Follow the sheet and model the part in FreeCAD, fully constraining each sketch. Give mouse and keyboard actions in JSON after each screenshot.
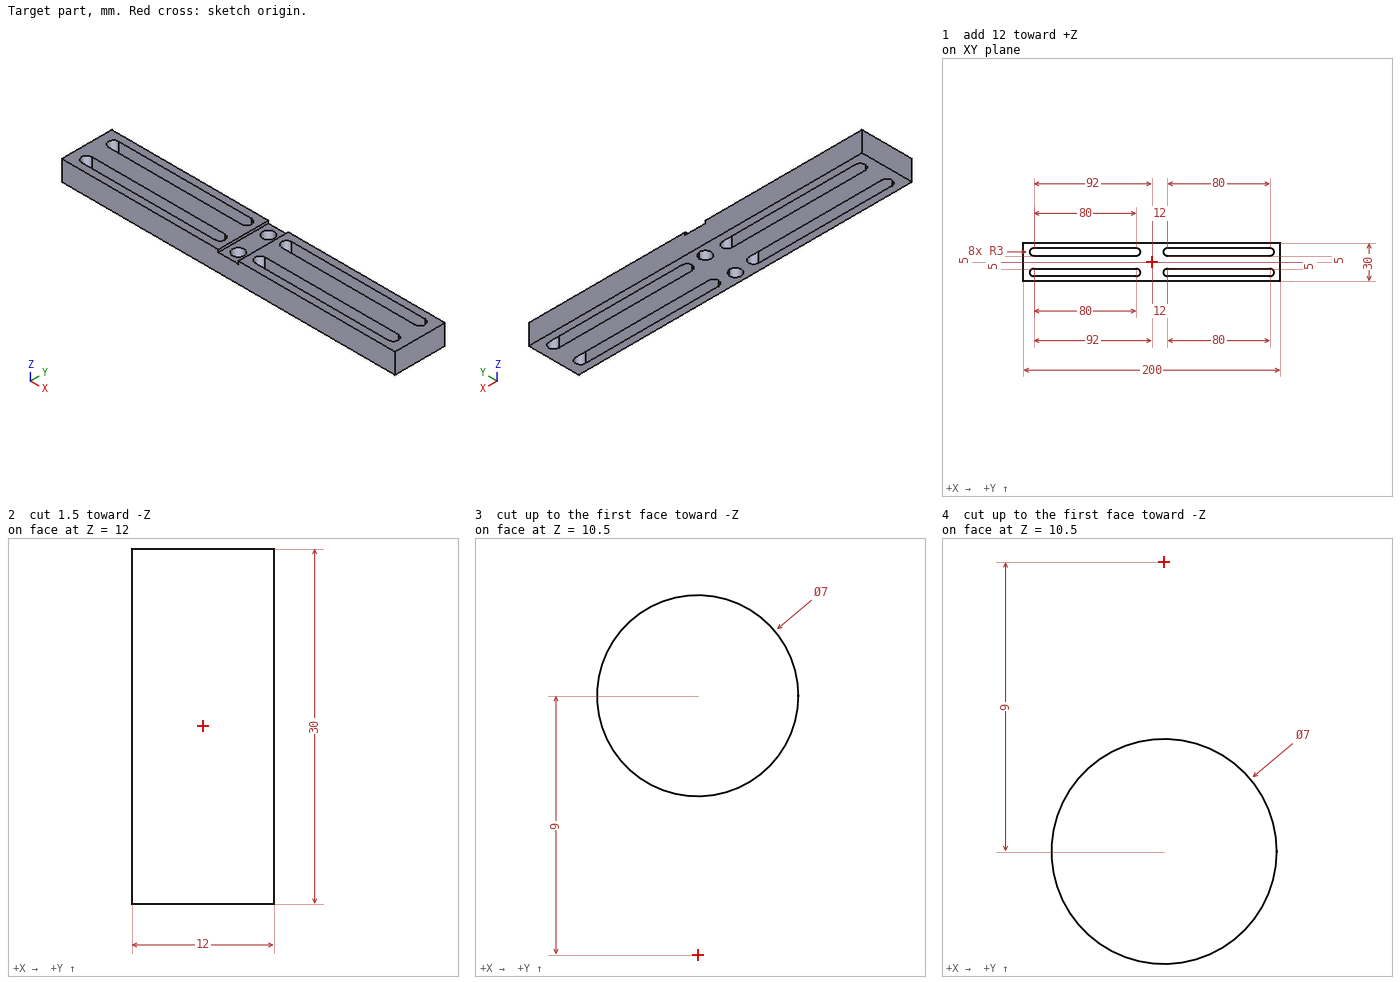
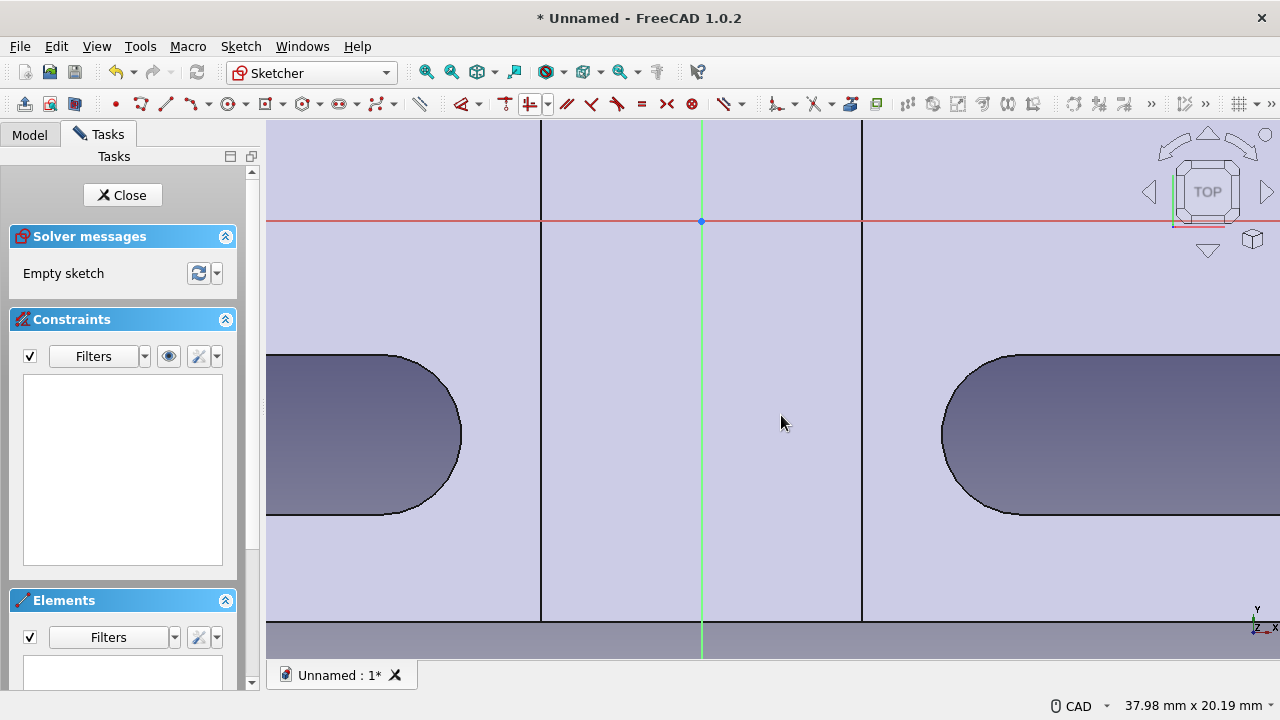
{"action": "left_click", "coordinate": [228, 104]}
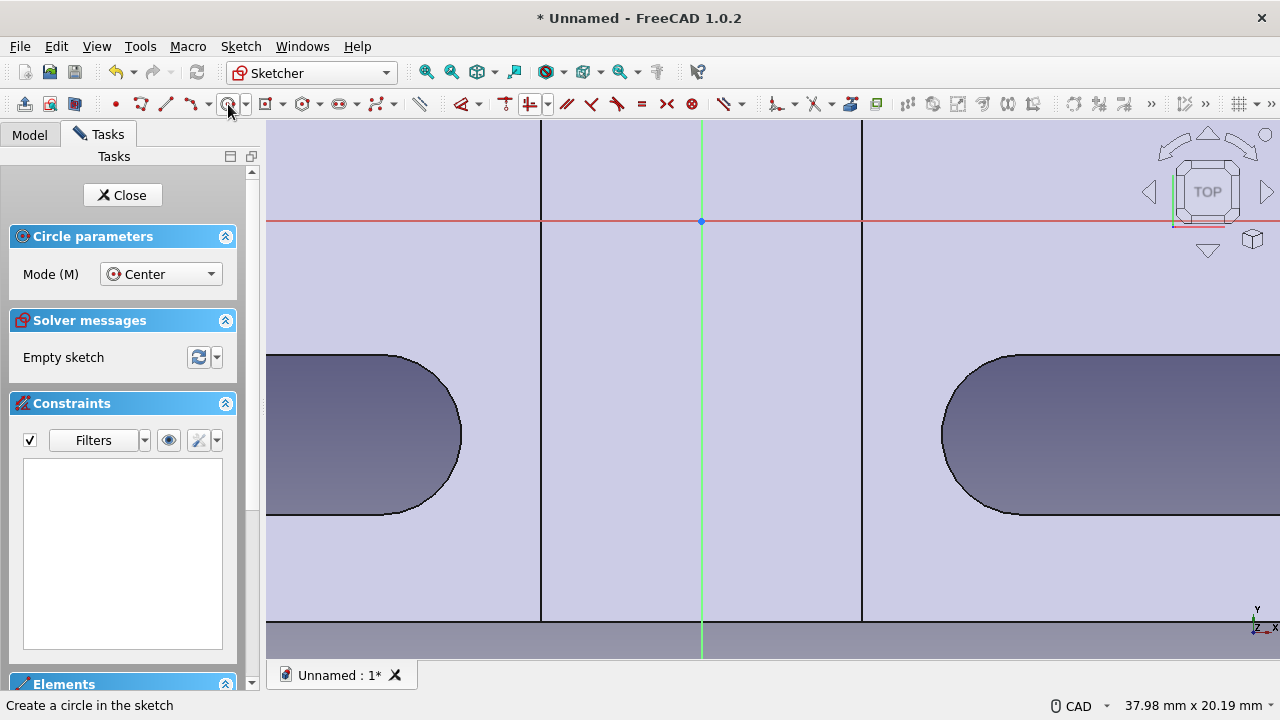
{"action": "left_click", "coordinate": [702, 461]}
{"action": "mouse_move", "coordinate": [768, 395]}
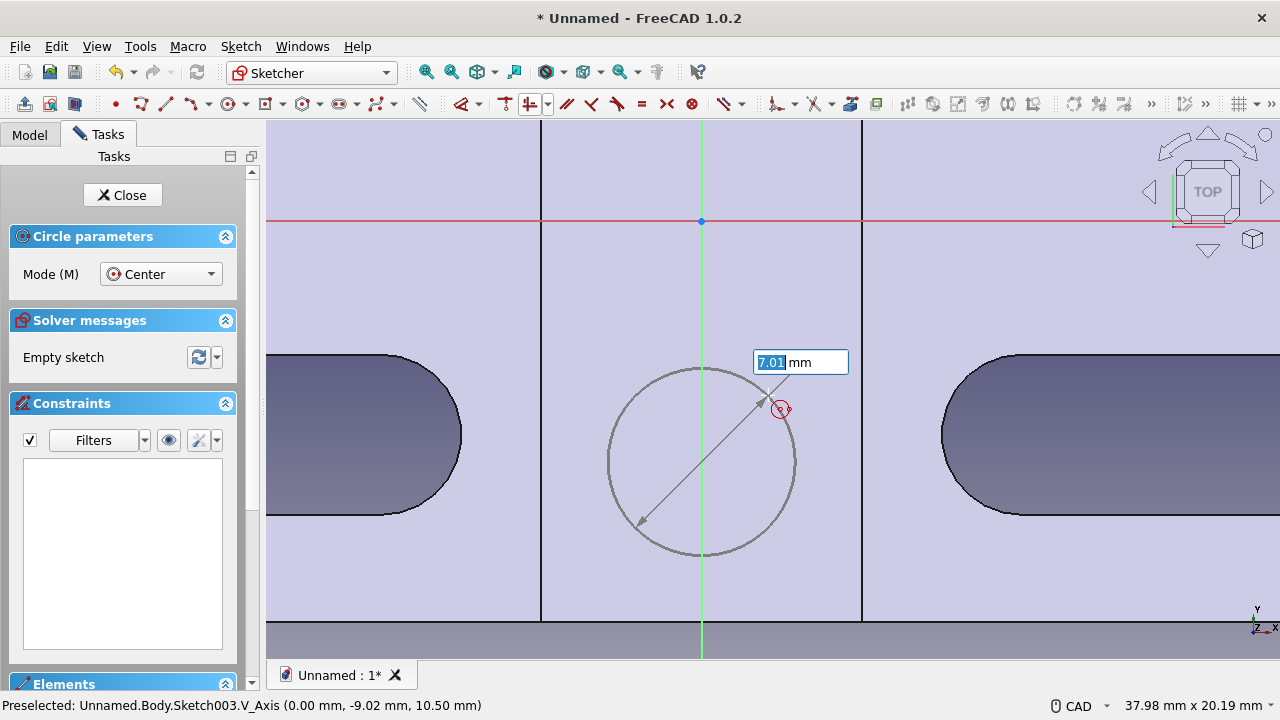
{"action": "type", "text": "7"}
{"action": "key", "text": "Return"}
{"action": "key", "text": "Escape"}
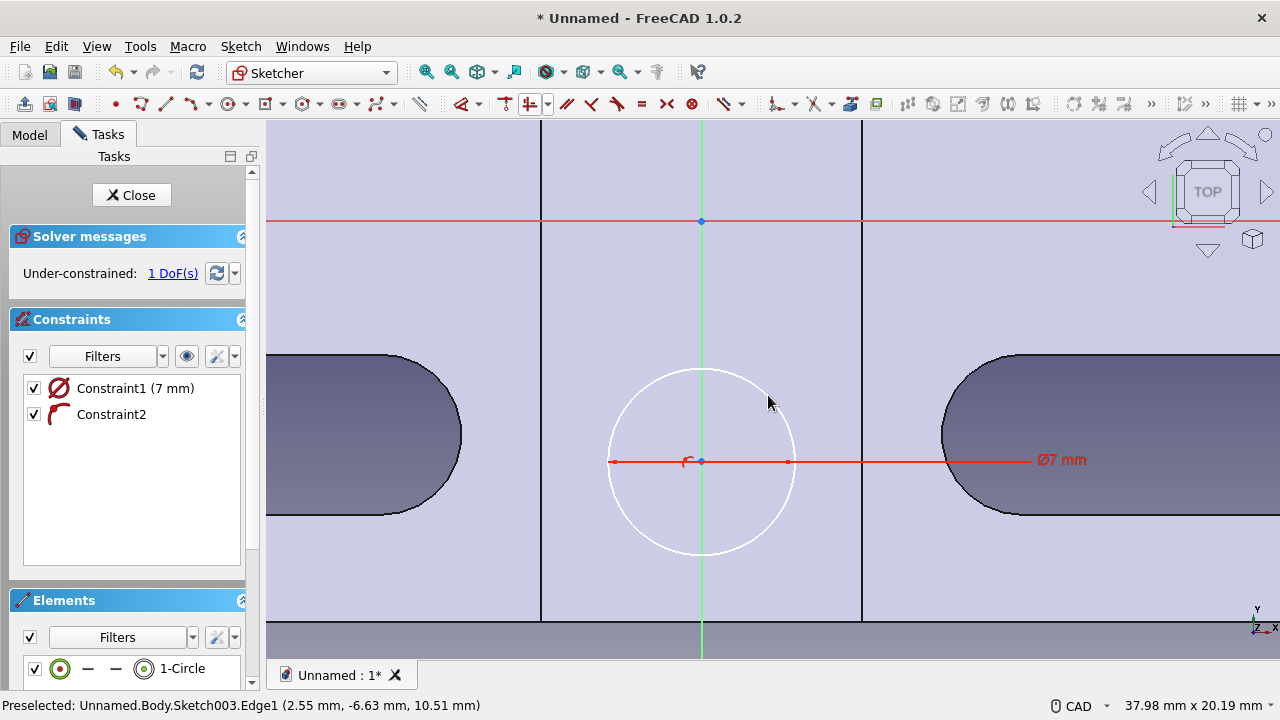
{"action": "left_click", "coordinate": [460, 104]}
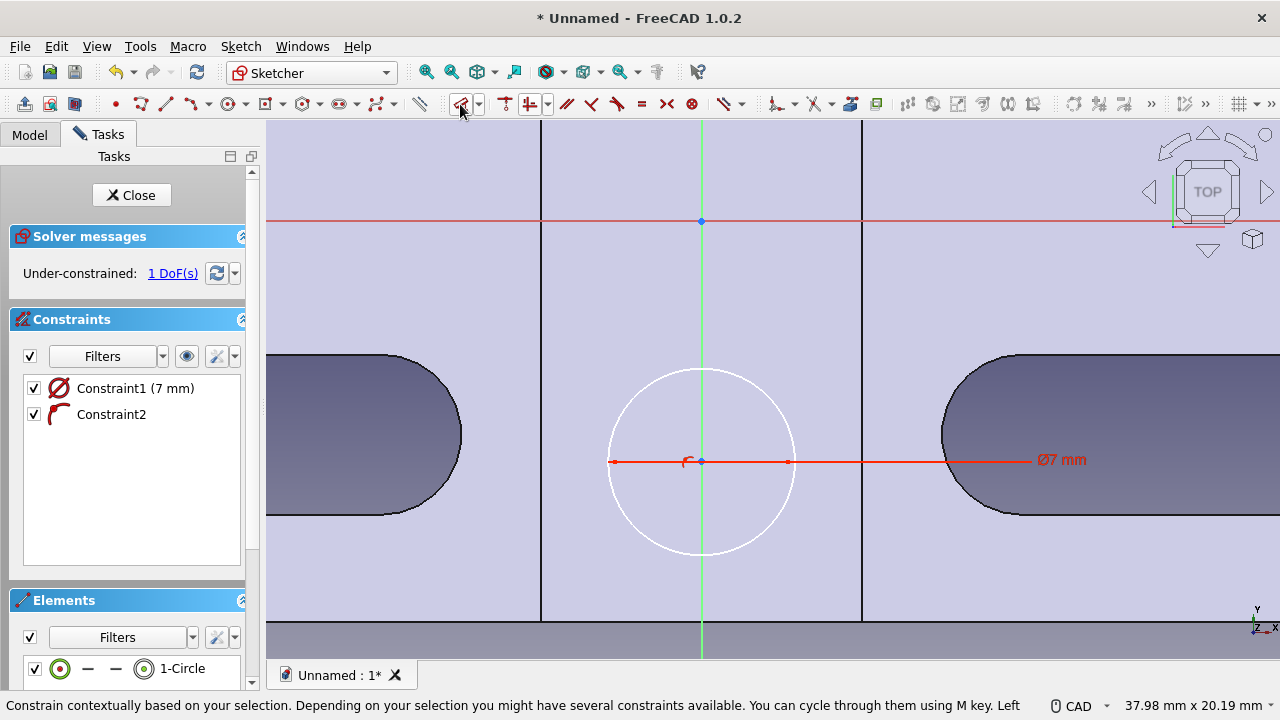
{"action": "left_click", "coordinate": [702, 462]}
{"action": "left_click", "coordinate": [736, 342]}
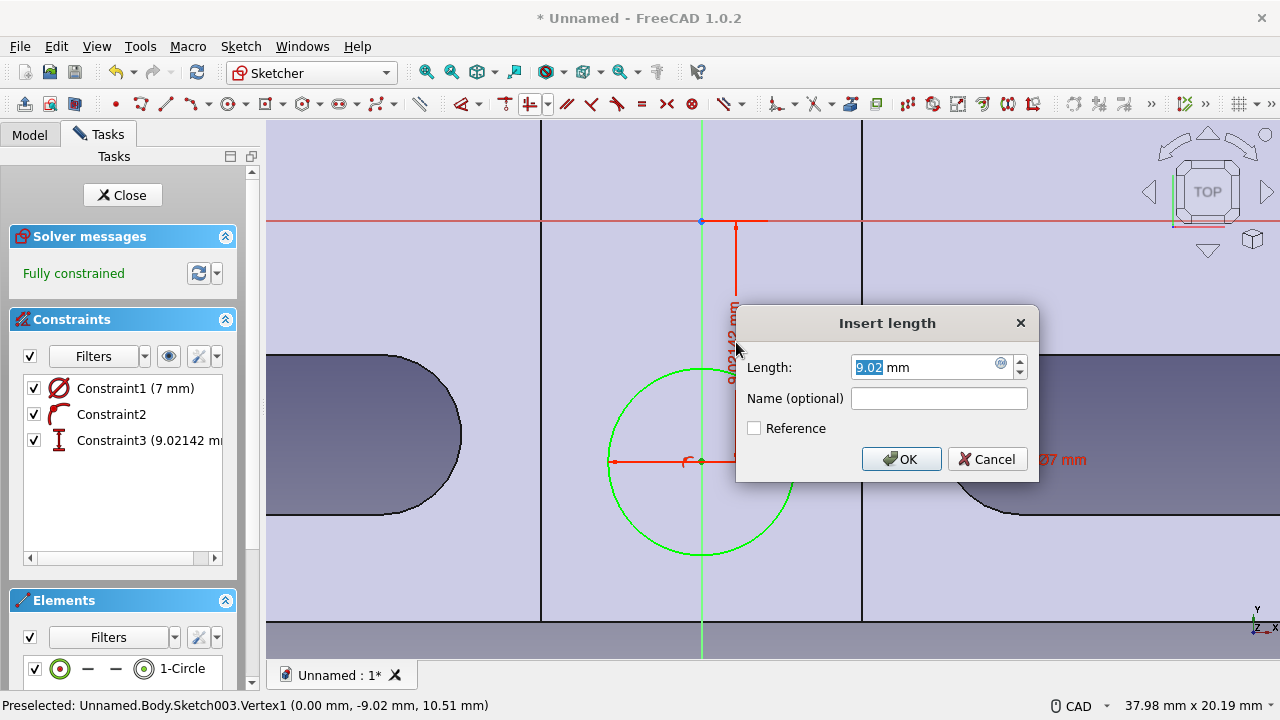
{"action": "type", "text": "9"}
{"action": "key", "text": "Return"}
{"action": "key", "text": "Escape"}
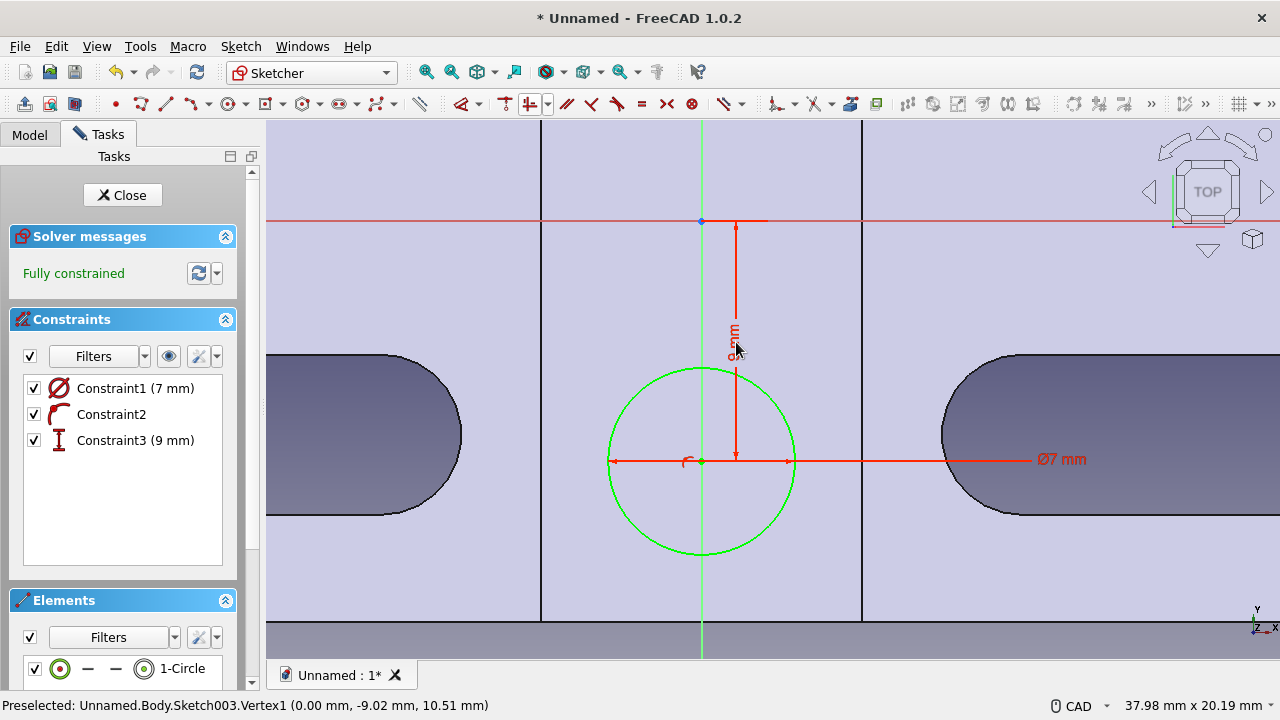
{"action": "left_click", "coordinate": [123, 195]}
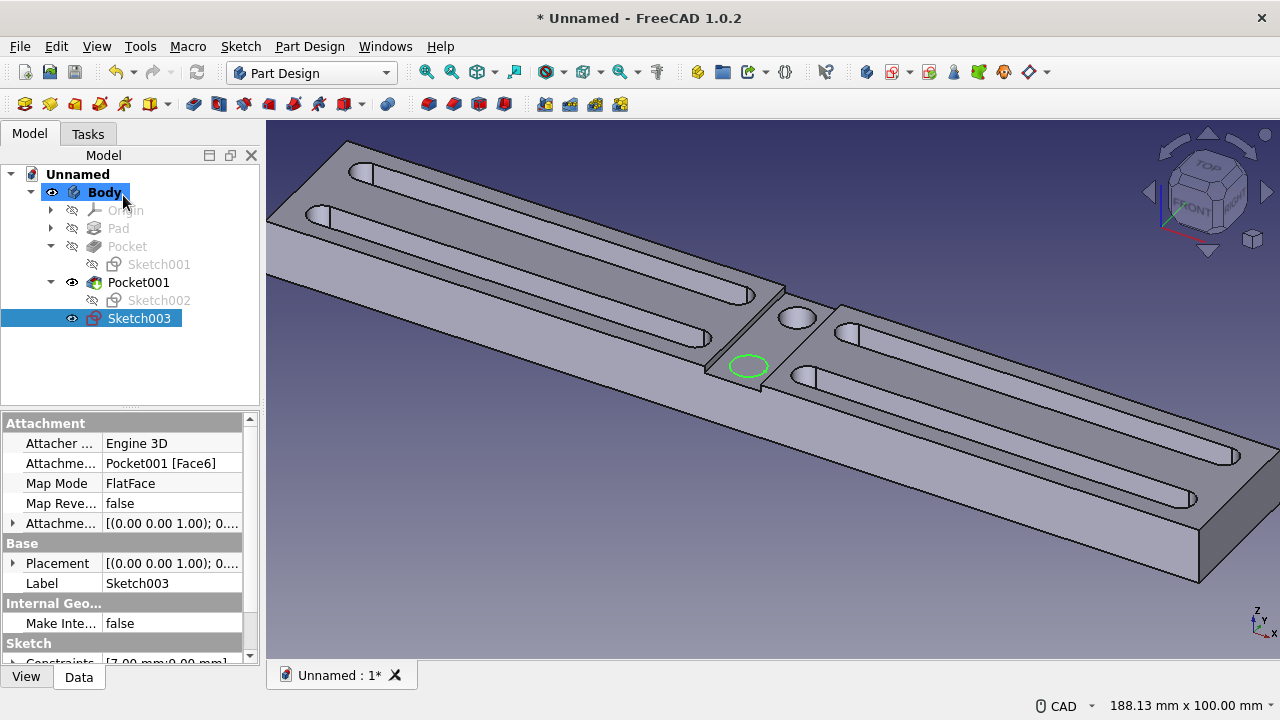
{"action": "left_click", "coordinate": [194, 104]}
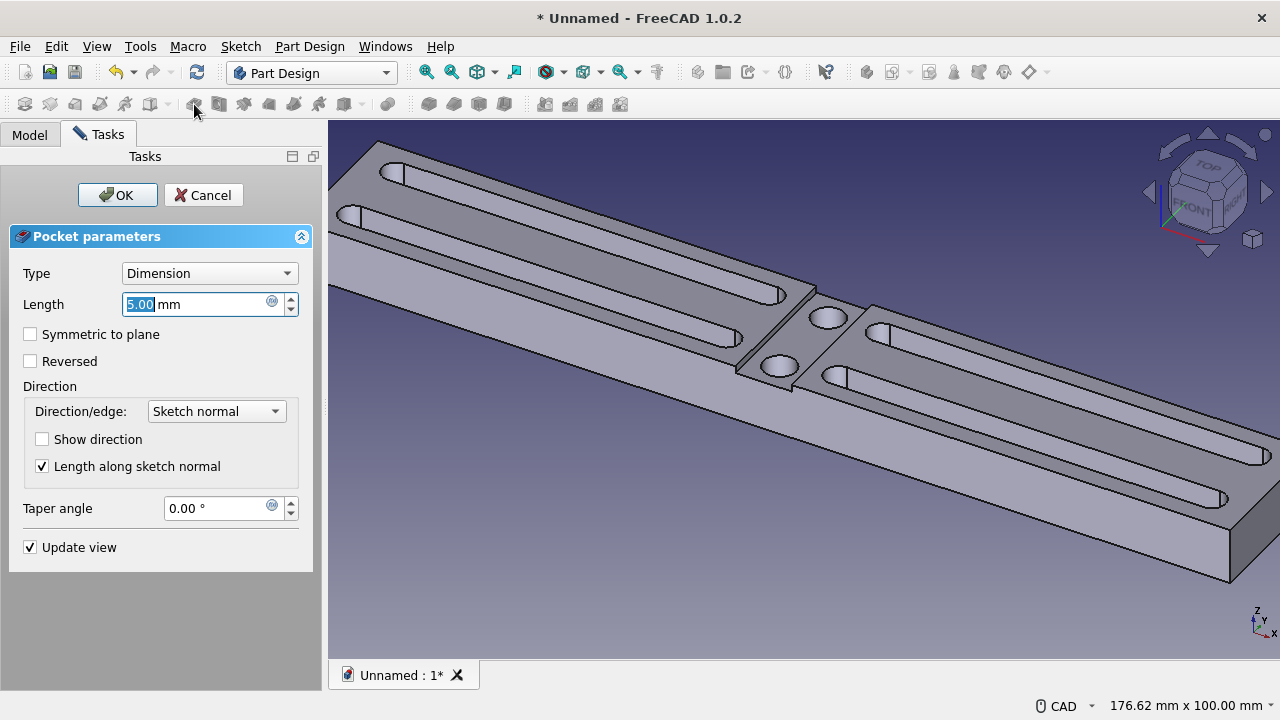
{"action": "left_click", "coordinate": [210, 274]}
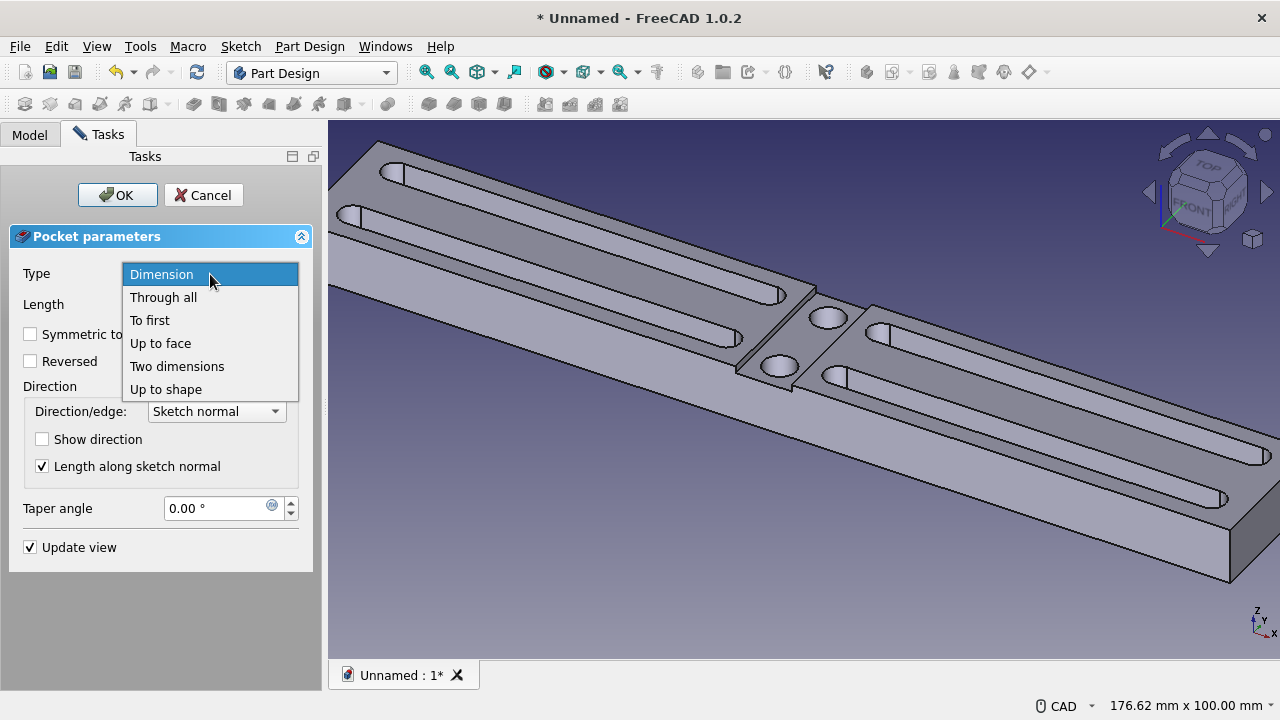
{"action": "left_click", "coordinate": [208, 320]}